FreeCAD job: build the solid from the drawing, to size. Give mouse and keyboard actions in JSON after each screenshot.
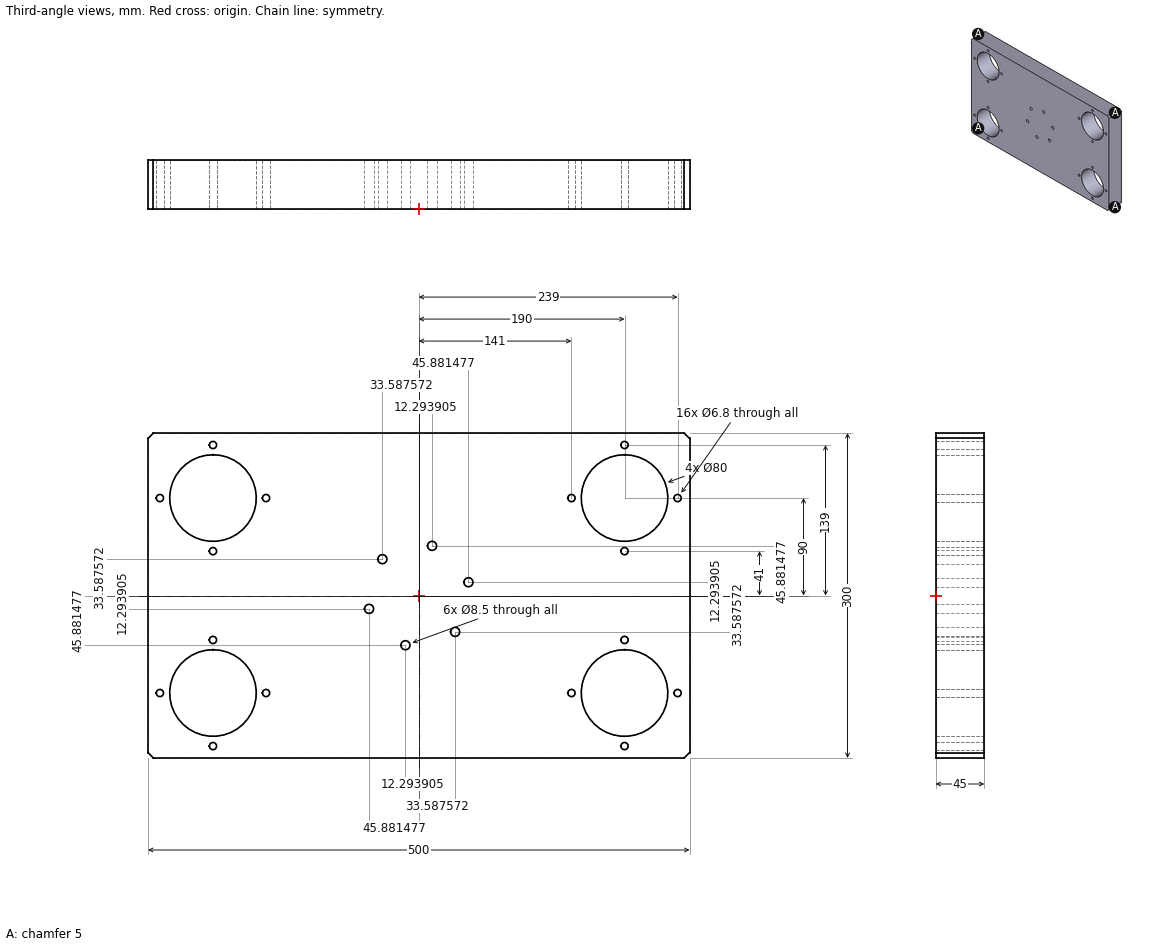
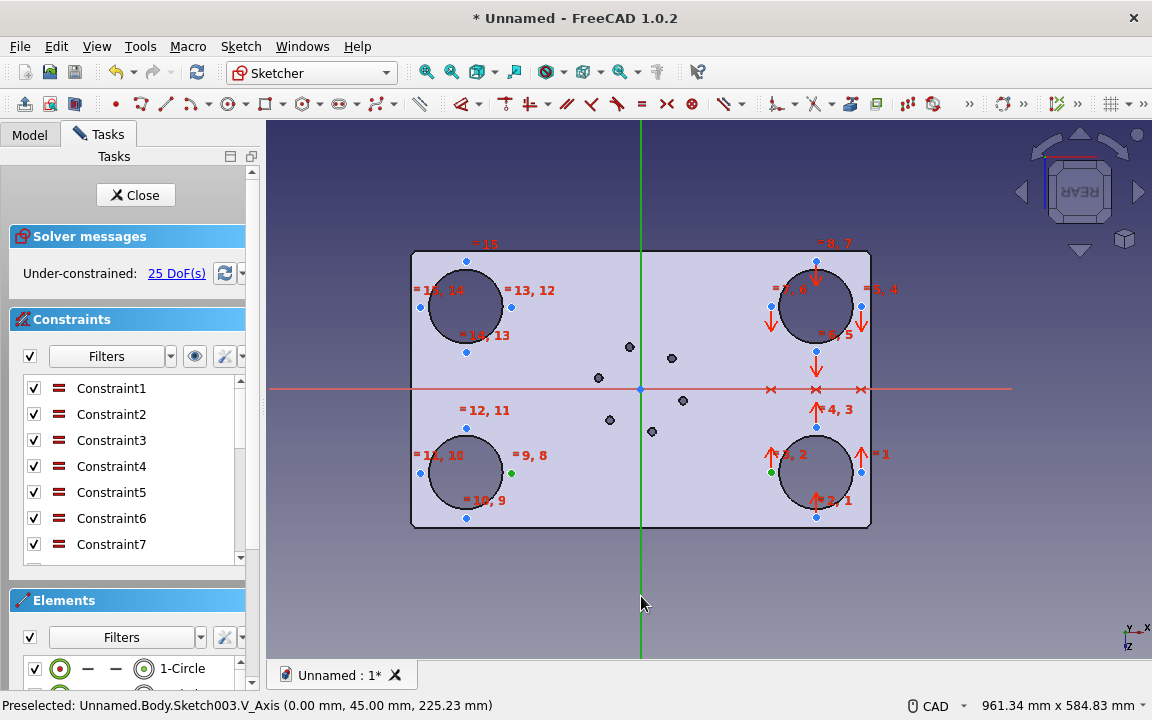
{"action": "left_click", "coordinate": [667, 104]}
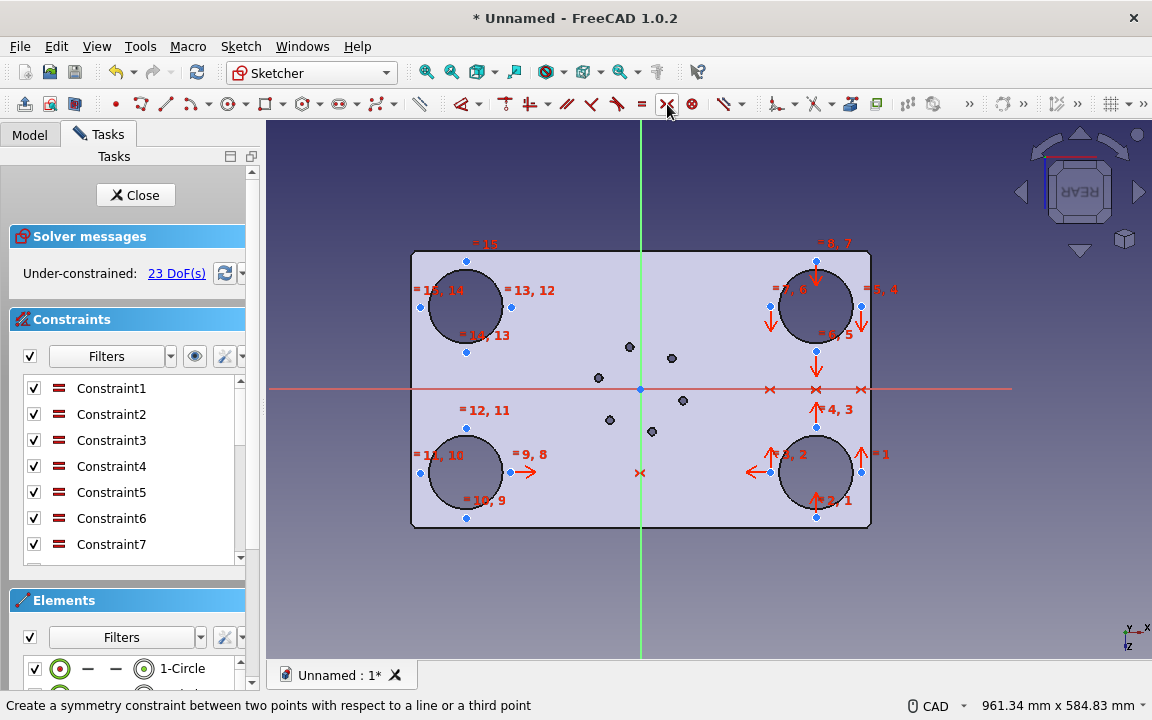
{"action": "left_click", "coordinate": [816, 518]}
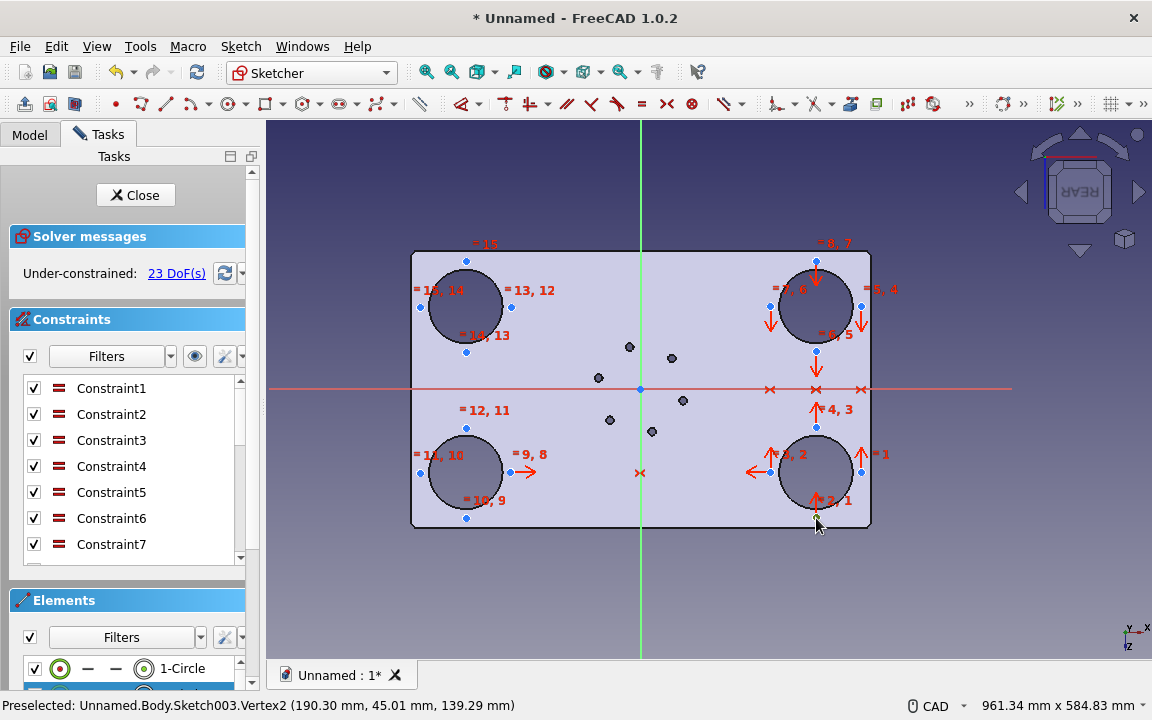
{"action": "left_click", "coordinate": [466, 518]}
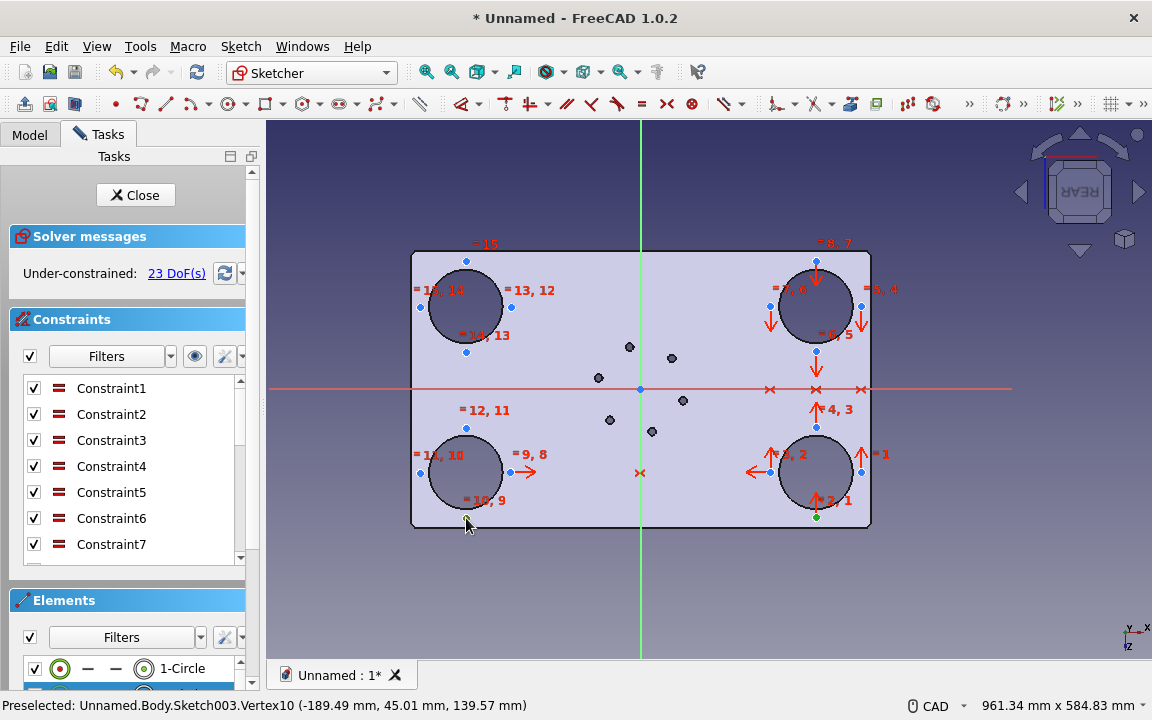
{"action": "left_click", "coordinate": [641, 596]}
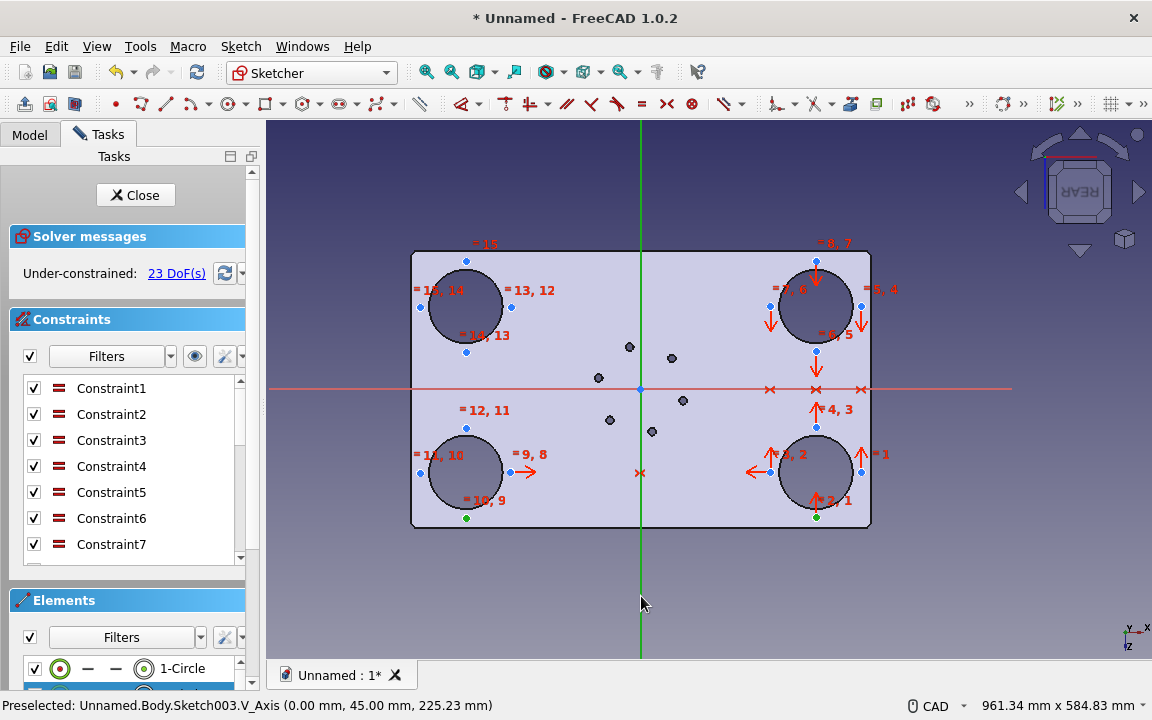
{"action": "left_click", "coordinate": [667, 104]}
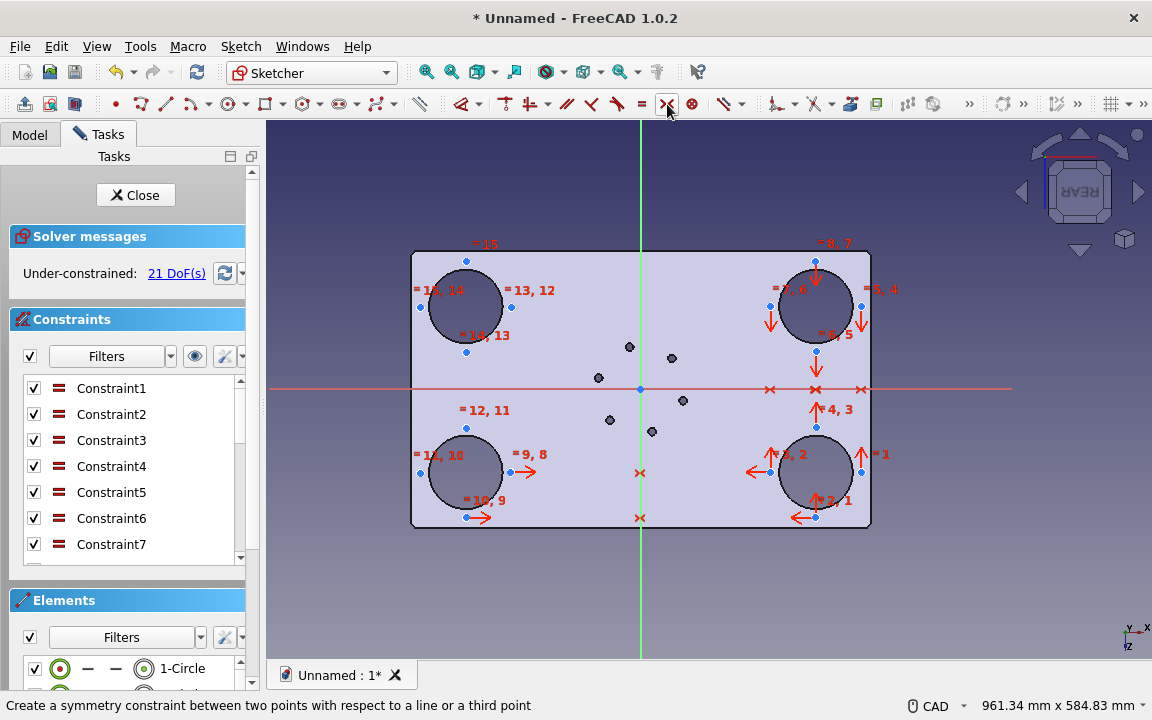
{"action": "left_click", "coordinate": [861, 472]}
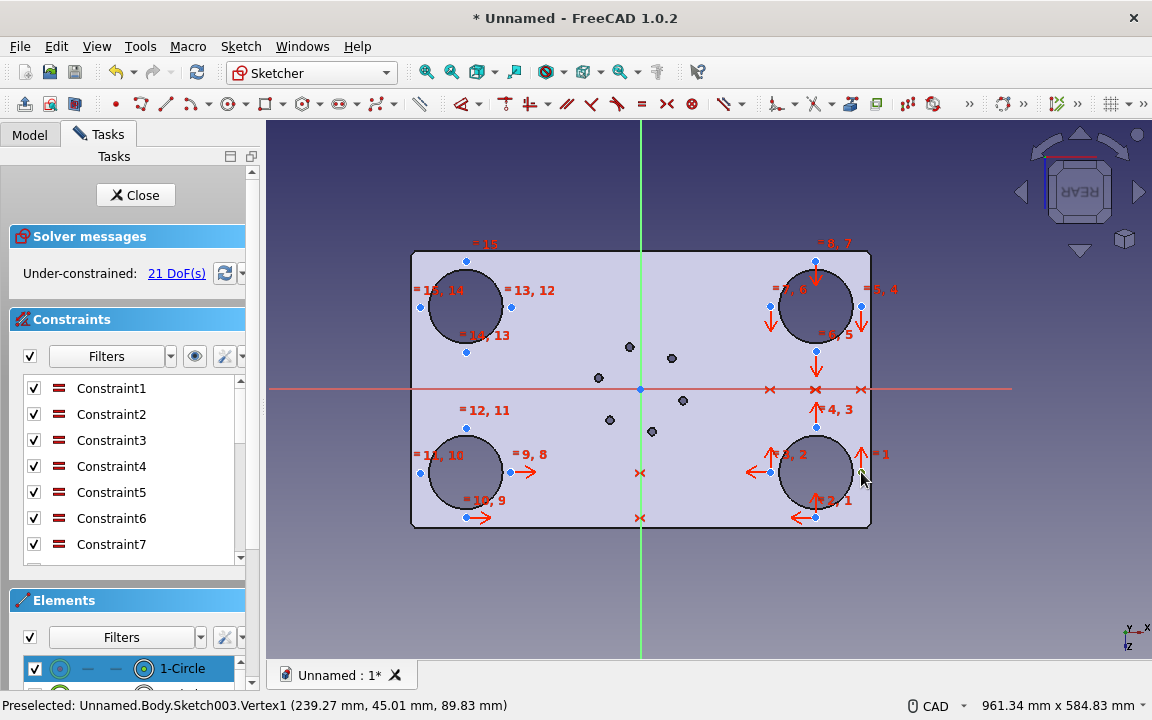
{"action": "left_click", "coordinate": [420, 473]}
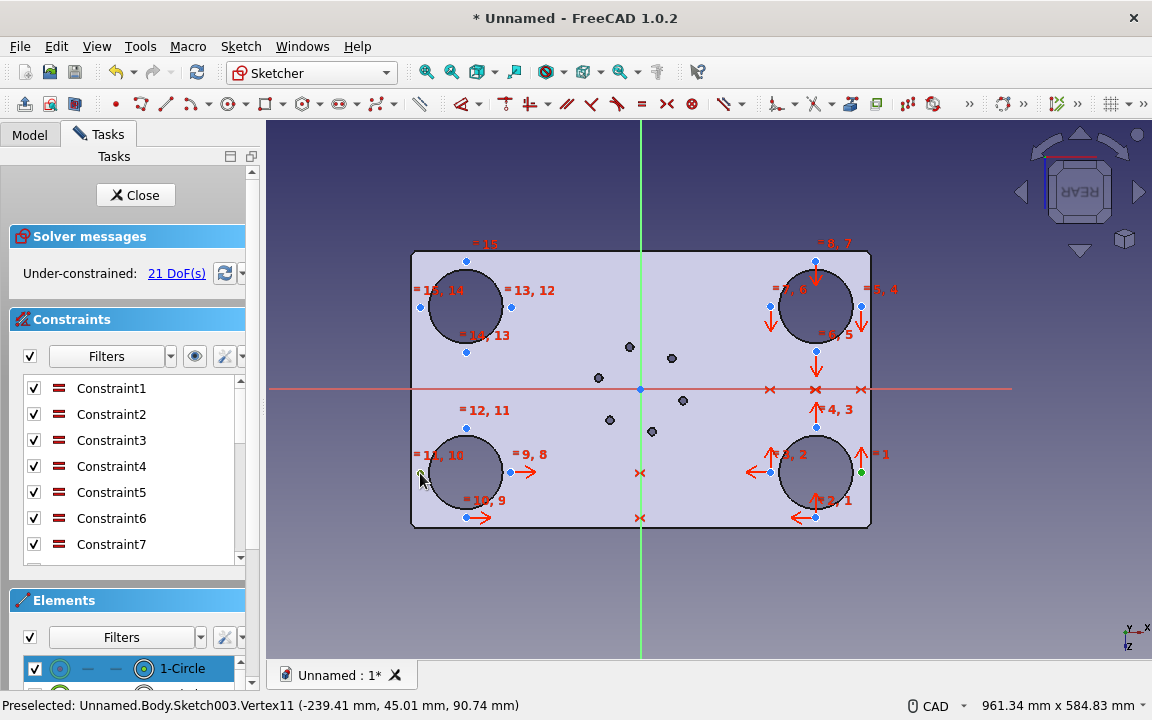
{"action": "left_click", "coordinate": [641, 596]}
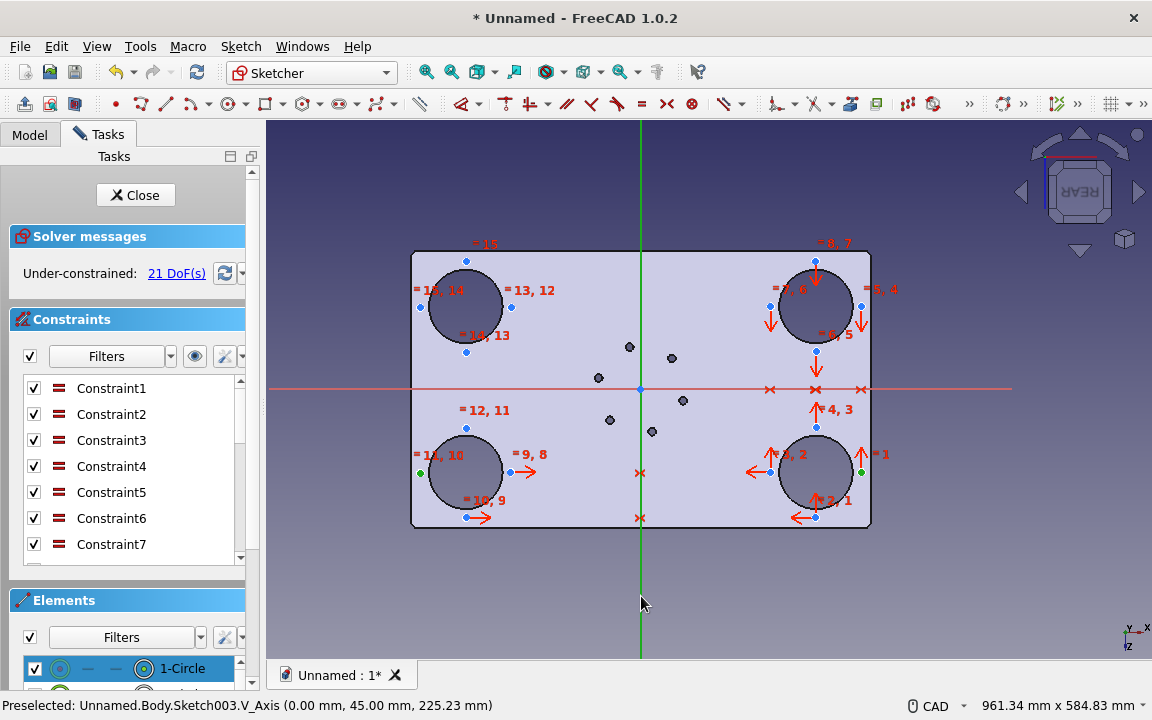
{"action": "left_click", "coordinate": [667, 104]}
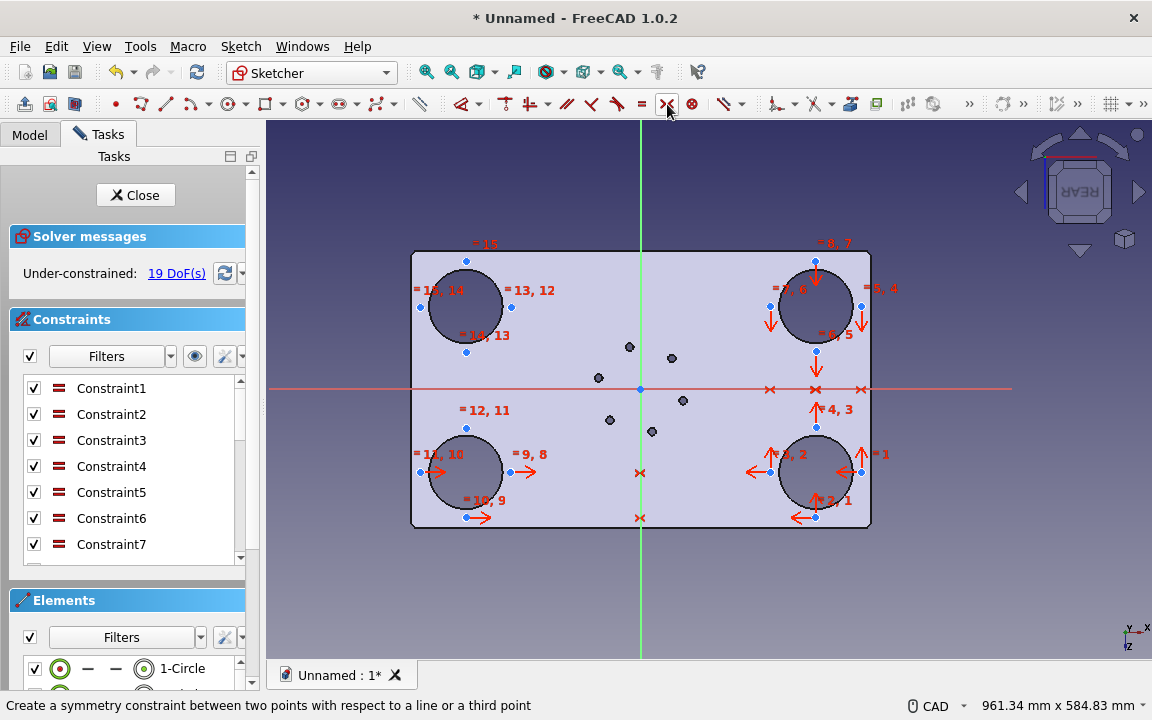
{"action": "left_click", "coordinate": [816, 427]}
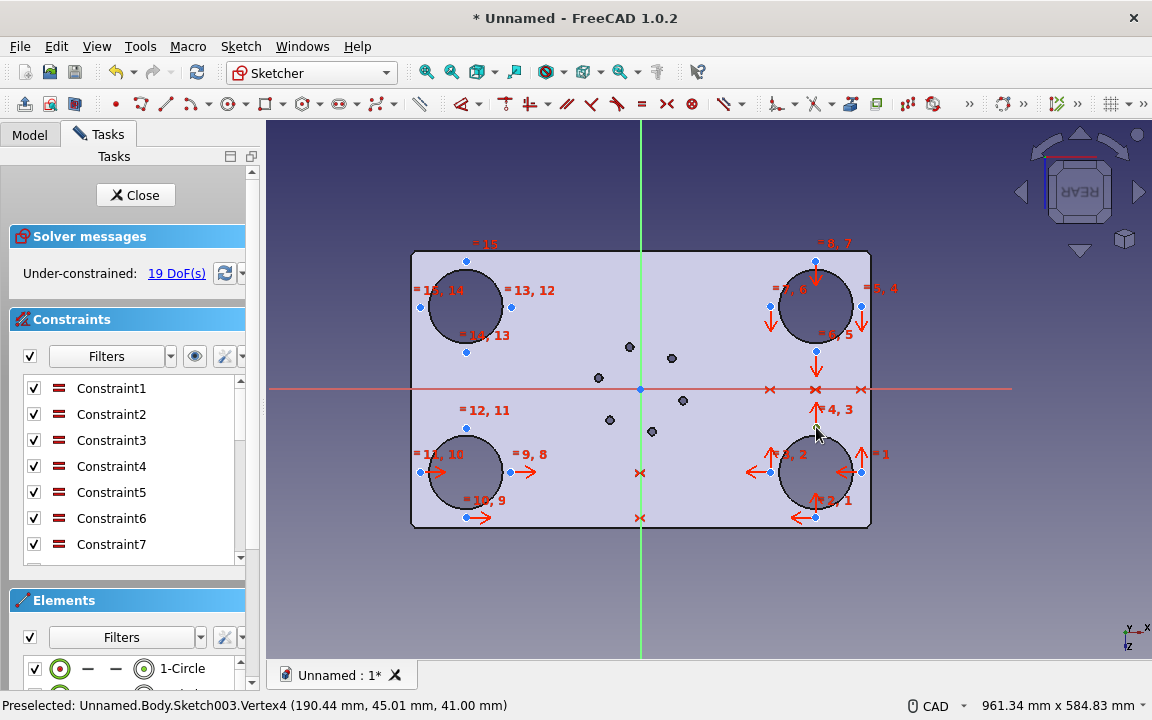
{"action": "left_click", "coordinate": [466, 428]}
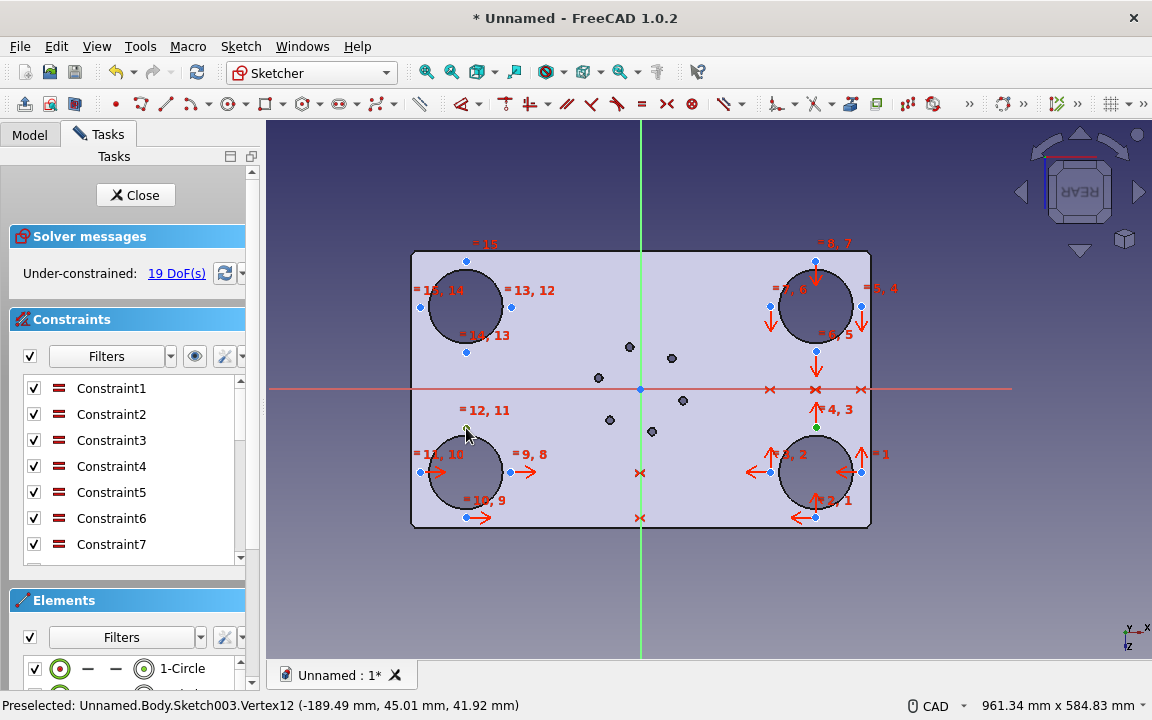
{"action": "left_click", "coordinate": [641, 596]}